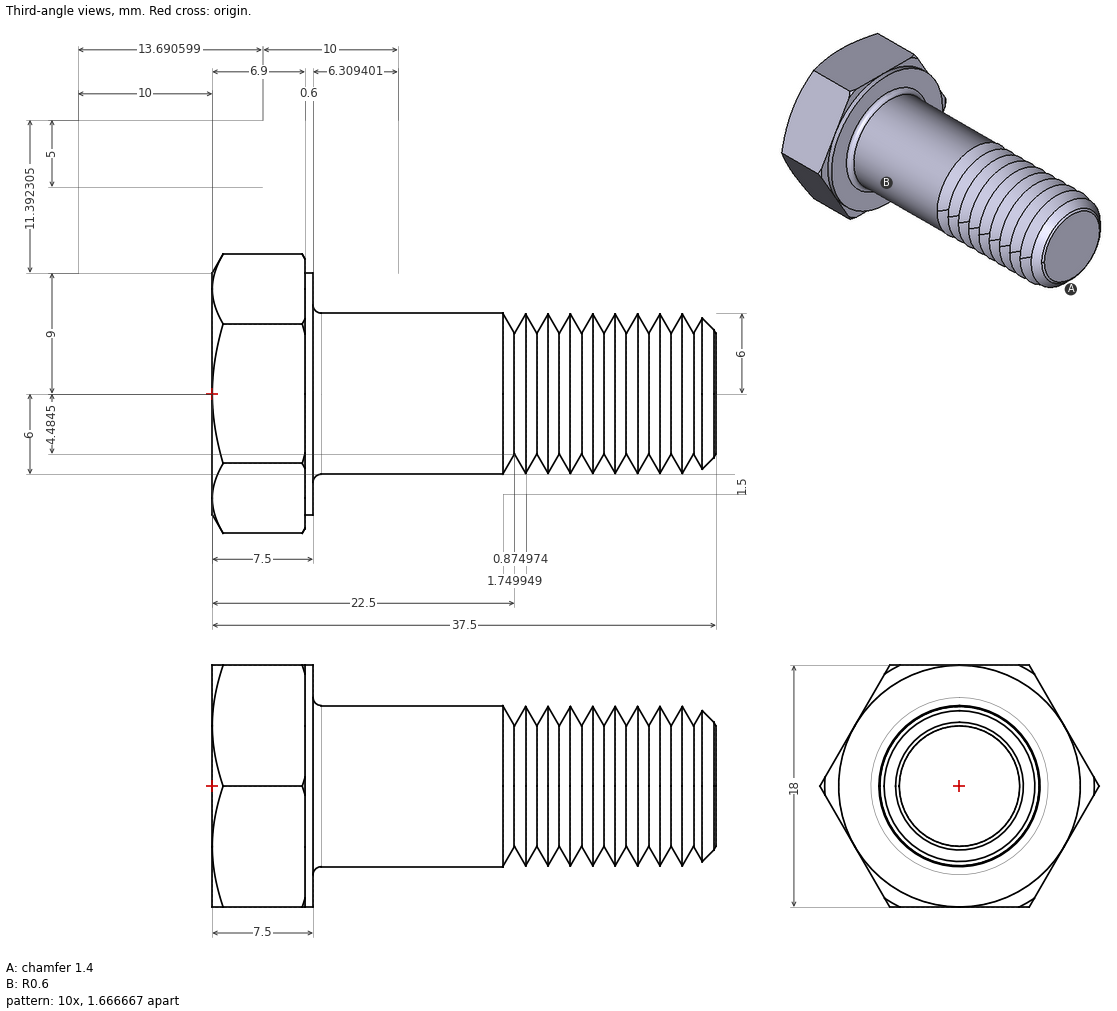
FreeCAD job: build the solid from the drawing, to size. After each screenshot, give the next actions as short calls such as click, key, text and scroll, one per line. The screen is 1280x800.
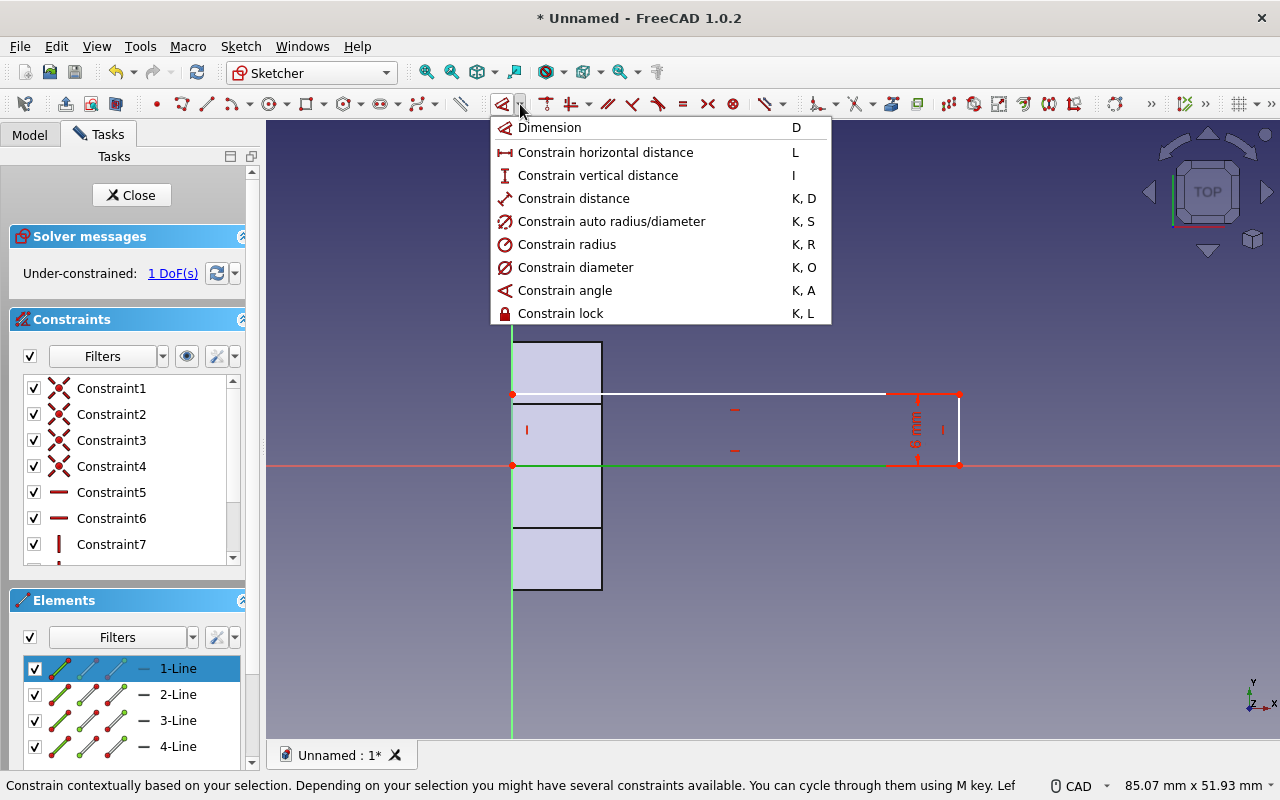
click(661, 152)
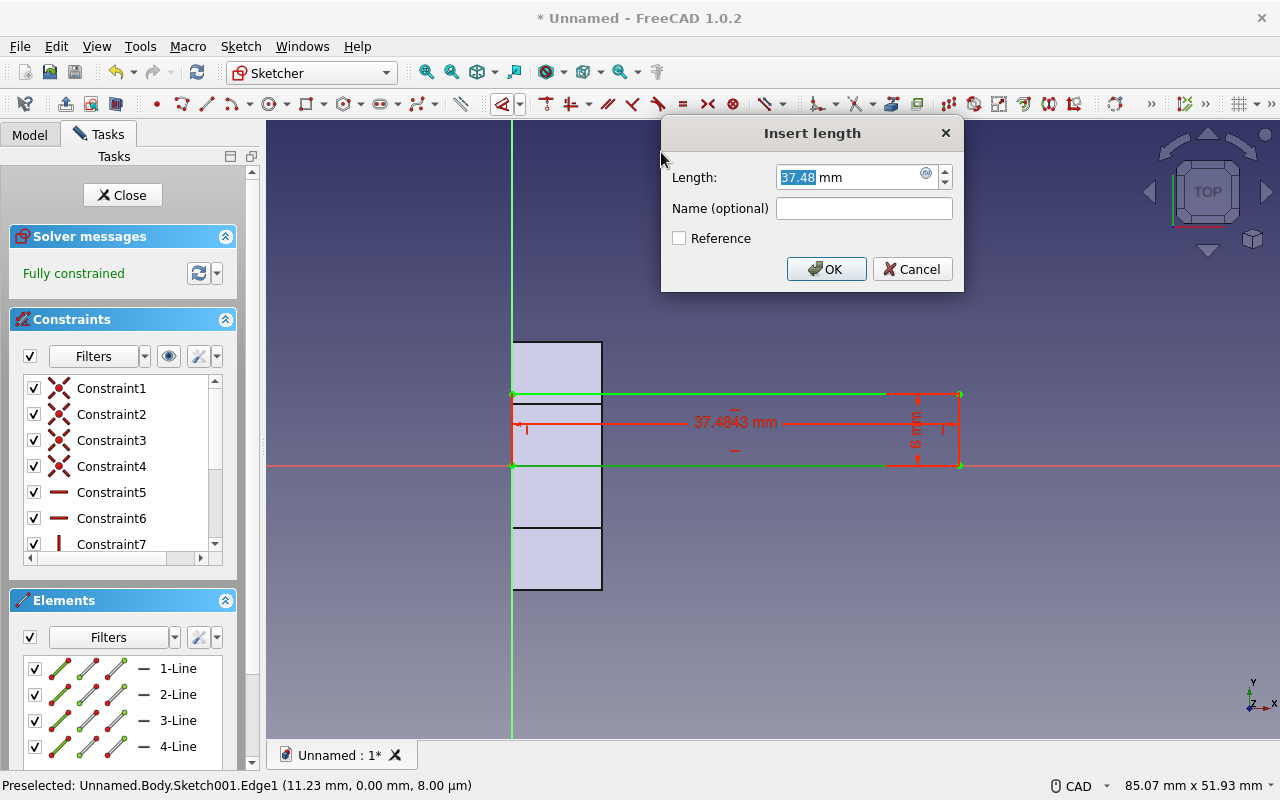
text(37.5)
key(Return)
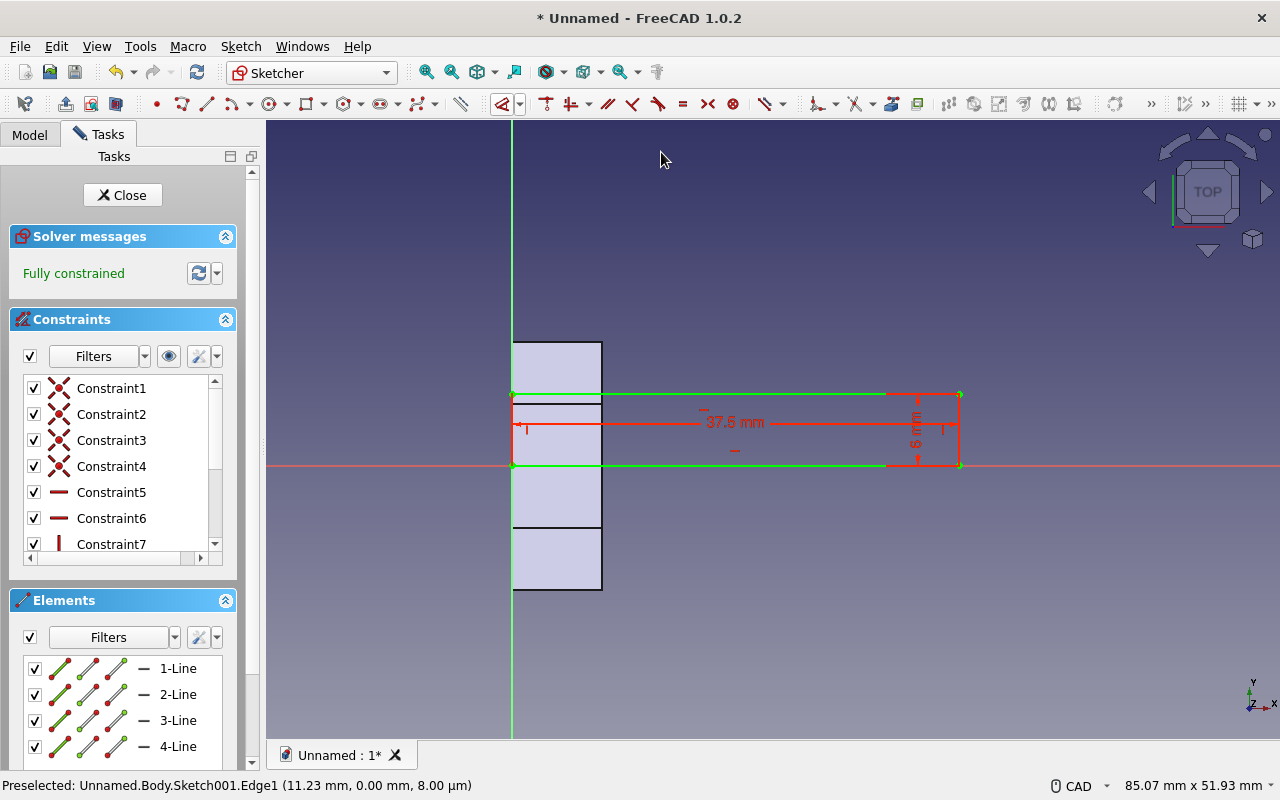
click(123, 195)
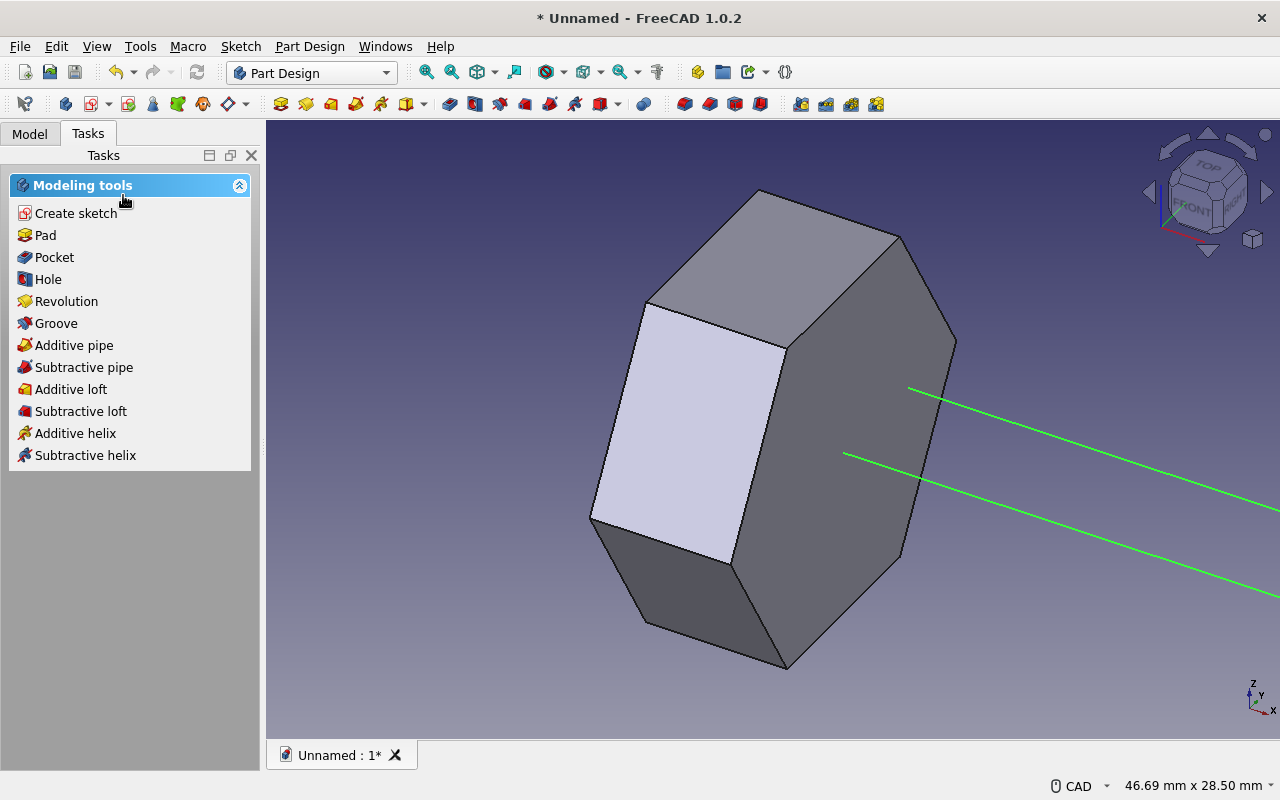
click(306, 104)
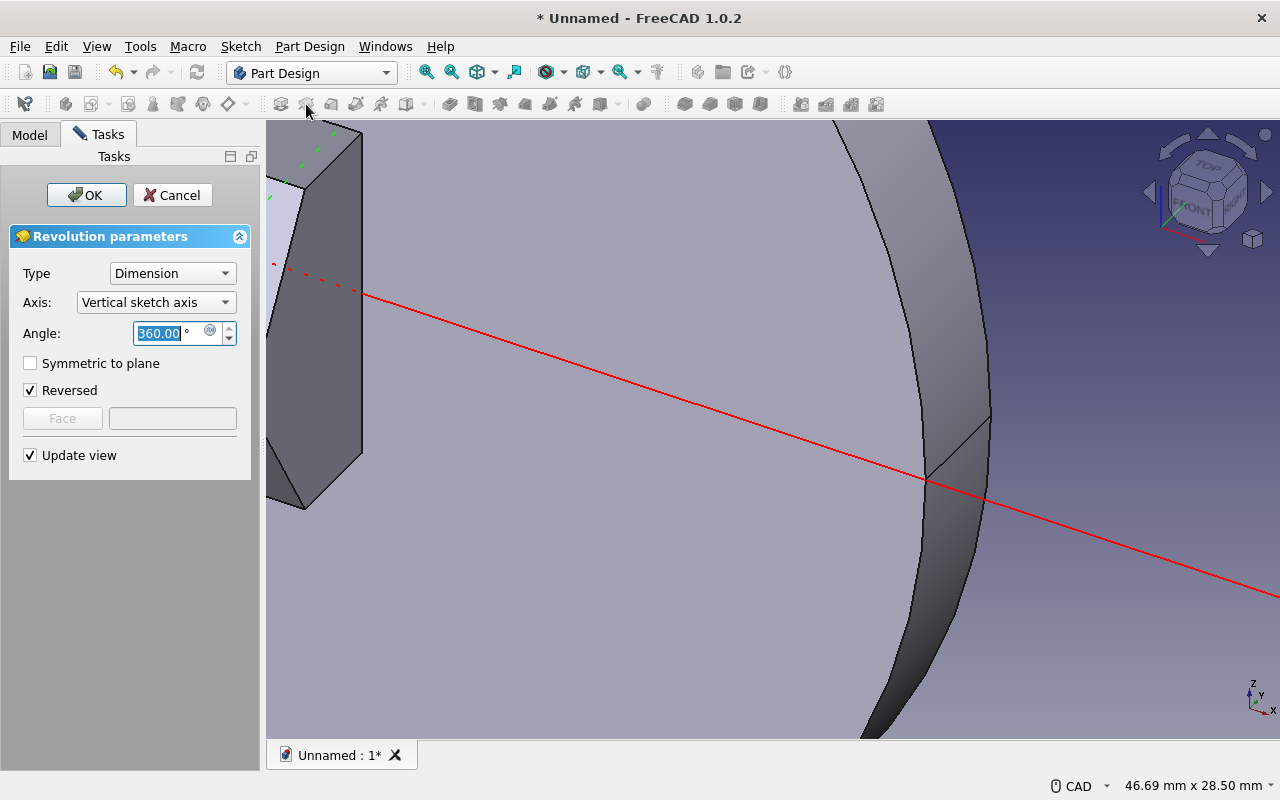
click(157, 302)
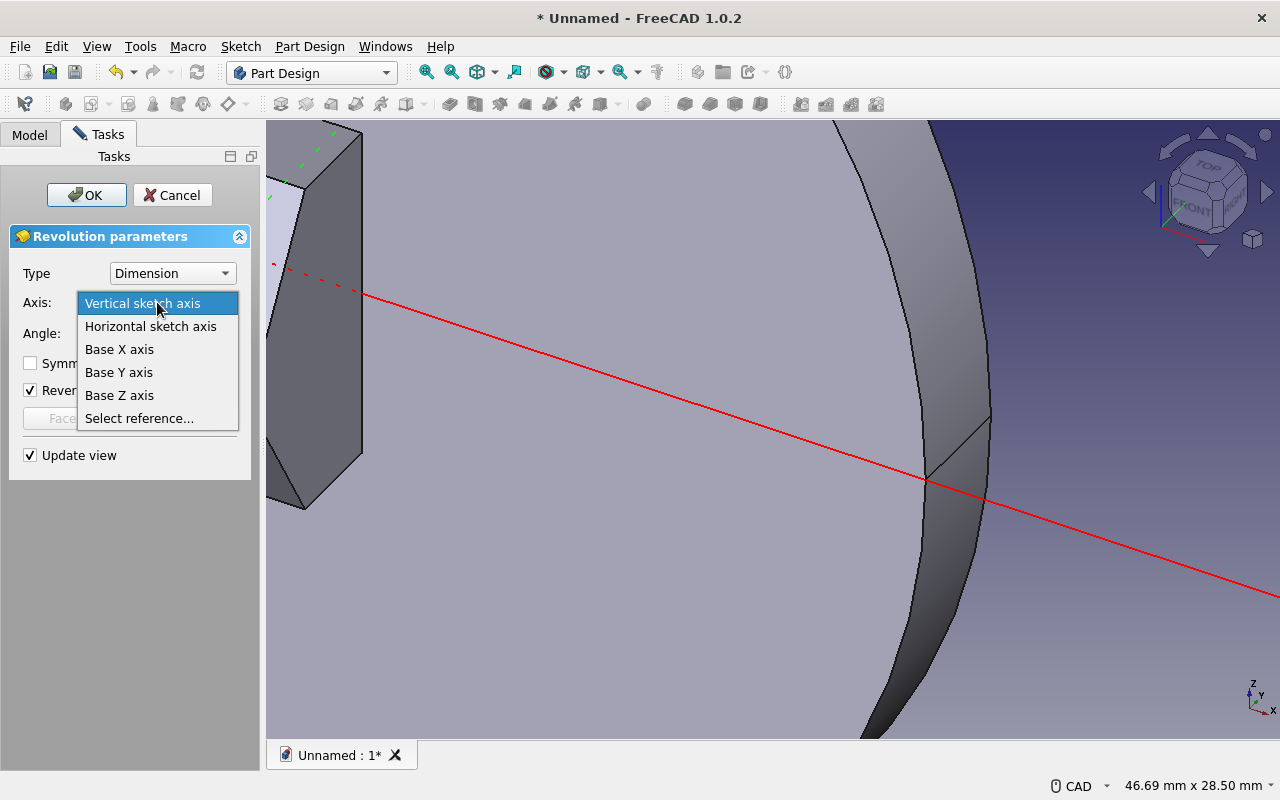
click(156, 326)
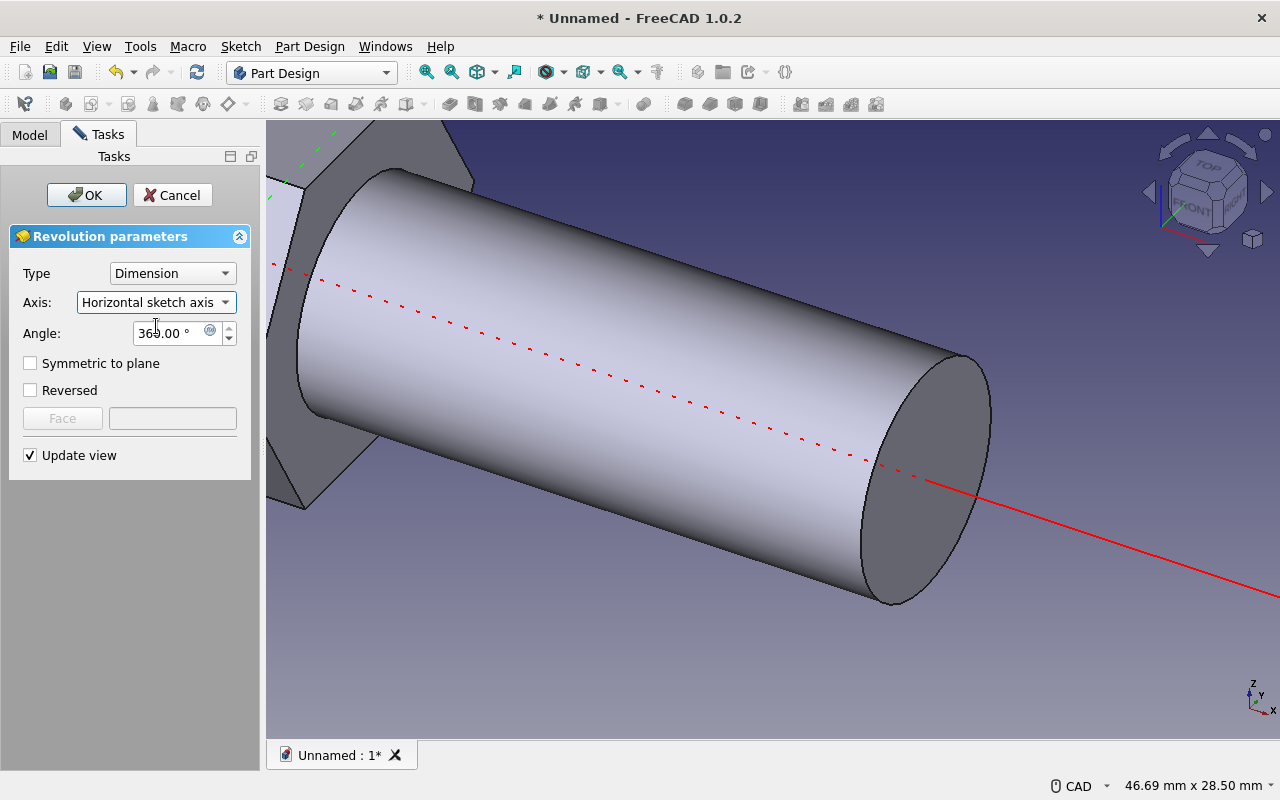
click(87, 195)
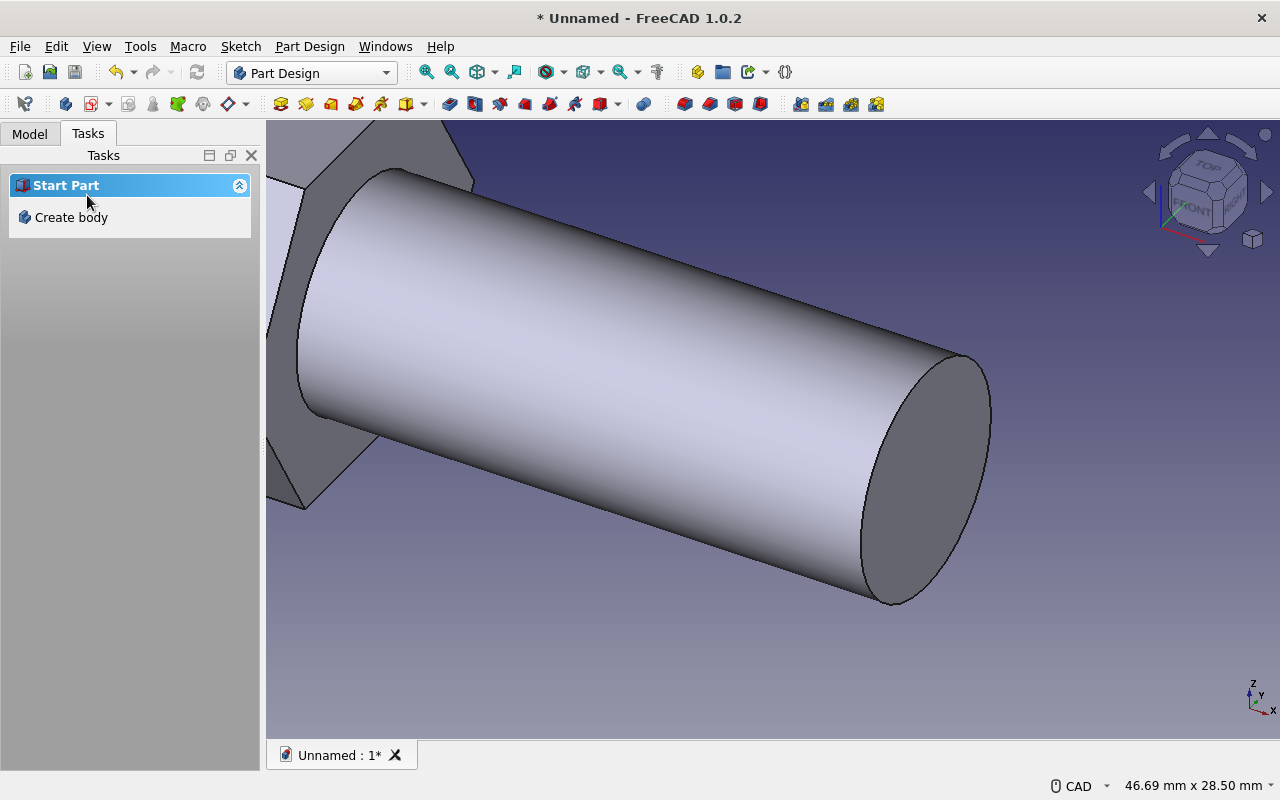
click(427, 72)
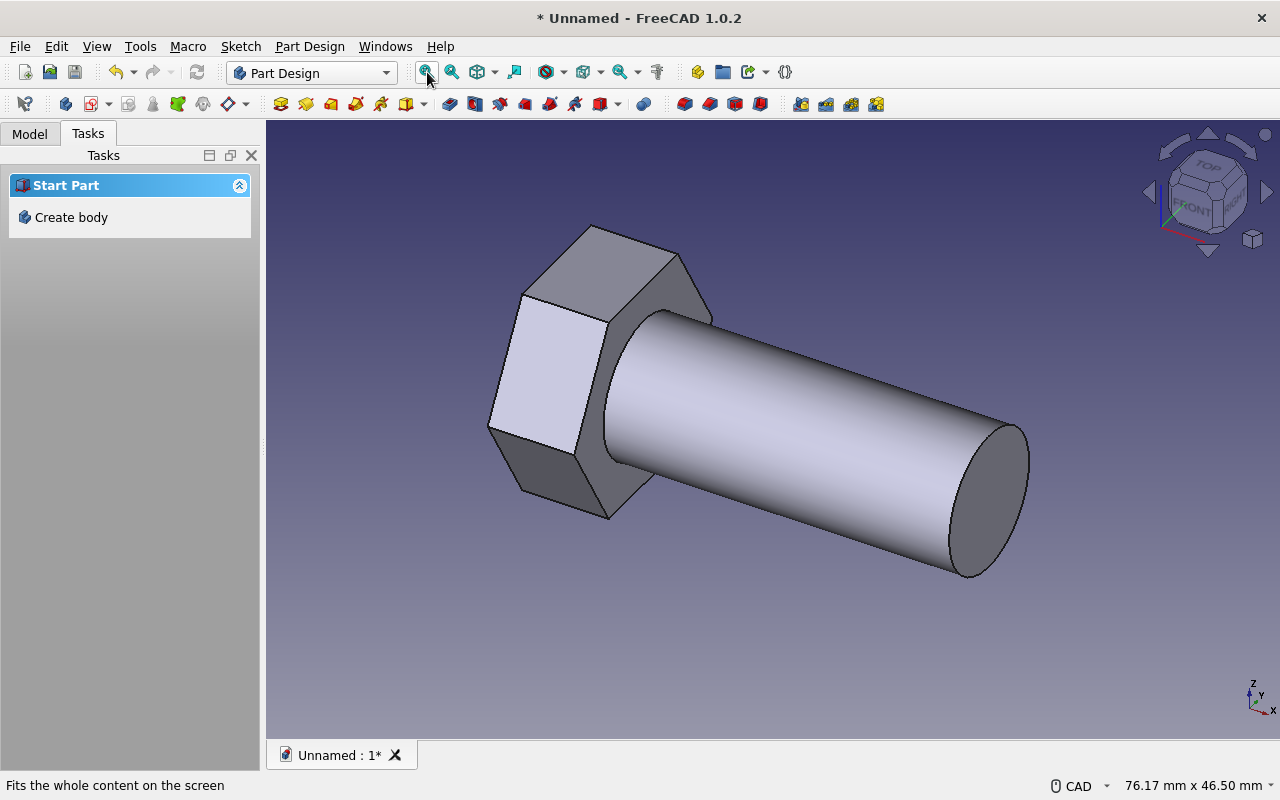
click(90, 104)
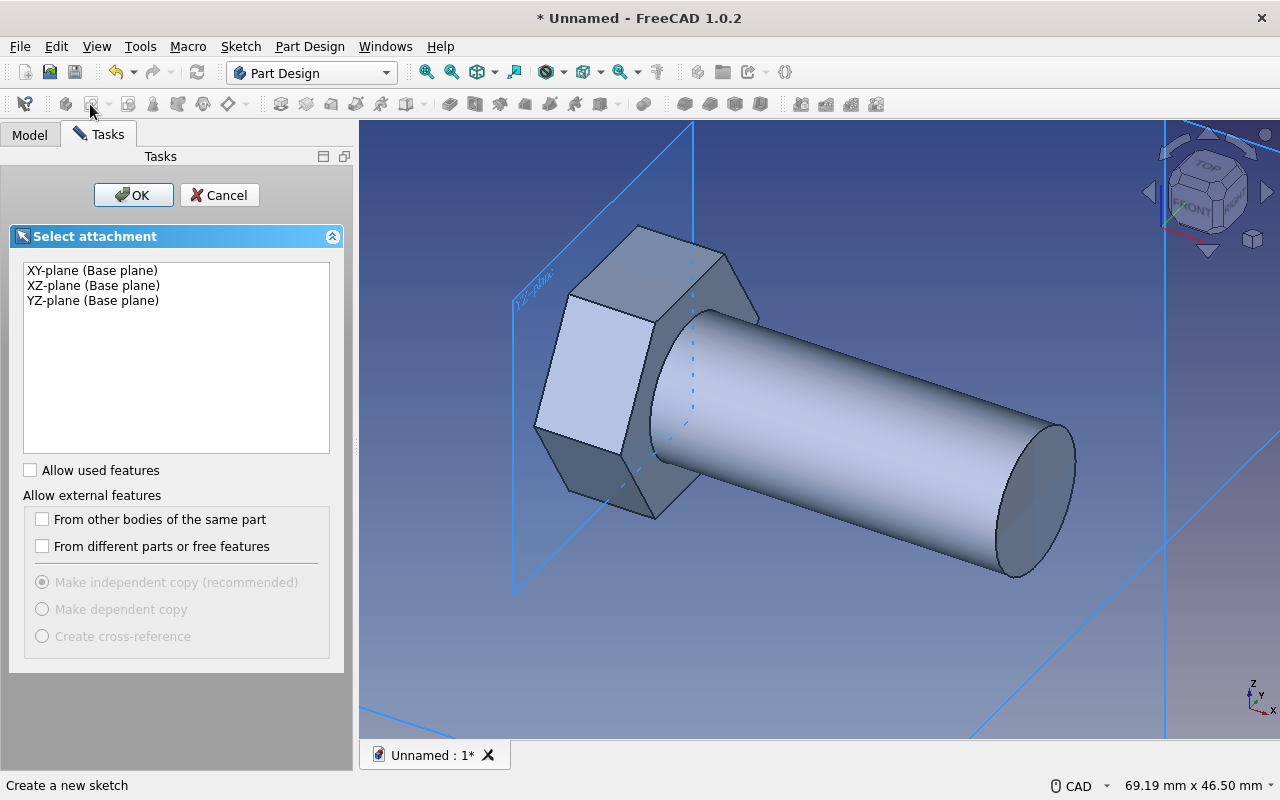
click(84, 270)